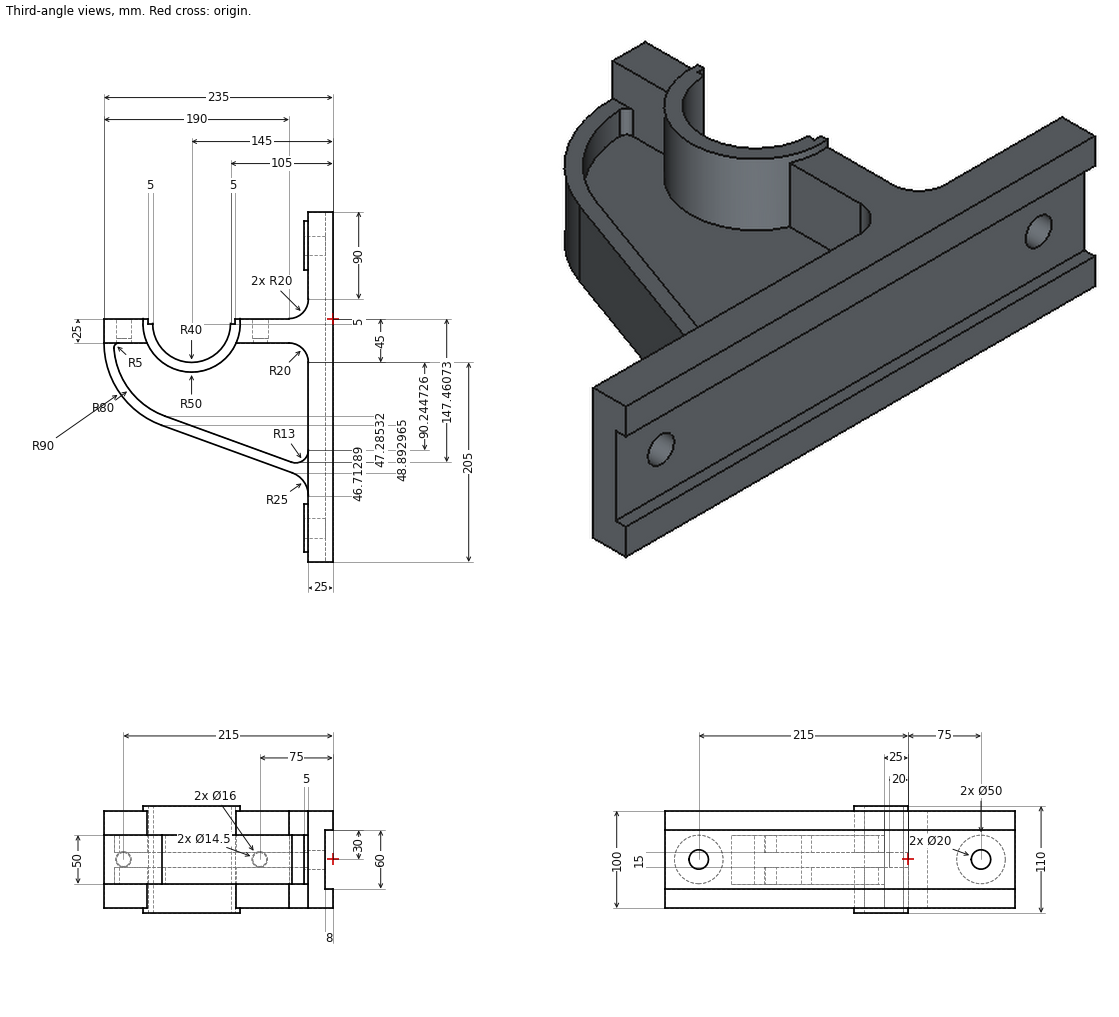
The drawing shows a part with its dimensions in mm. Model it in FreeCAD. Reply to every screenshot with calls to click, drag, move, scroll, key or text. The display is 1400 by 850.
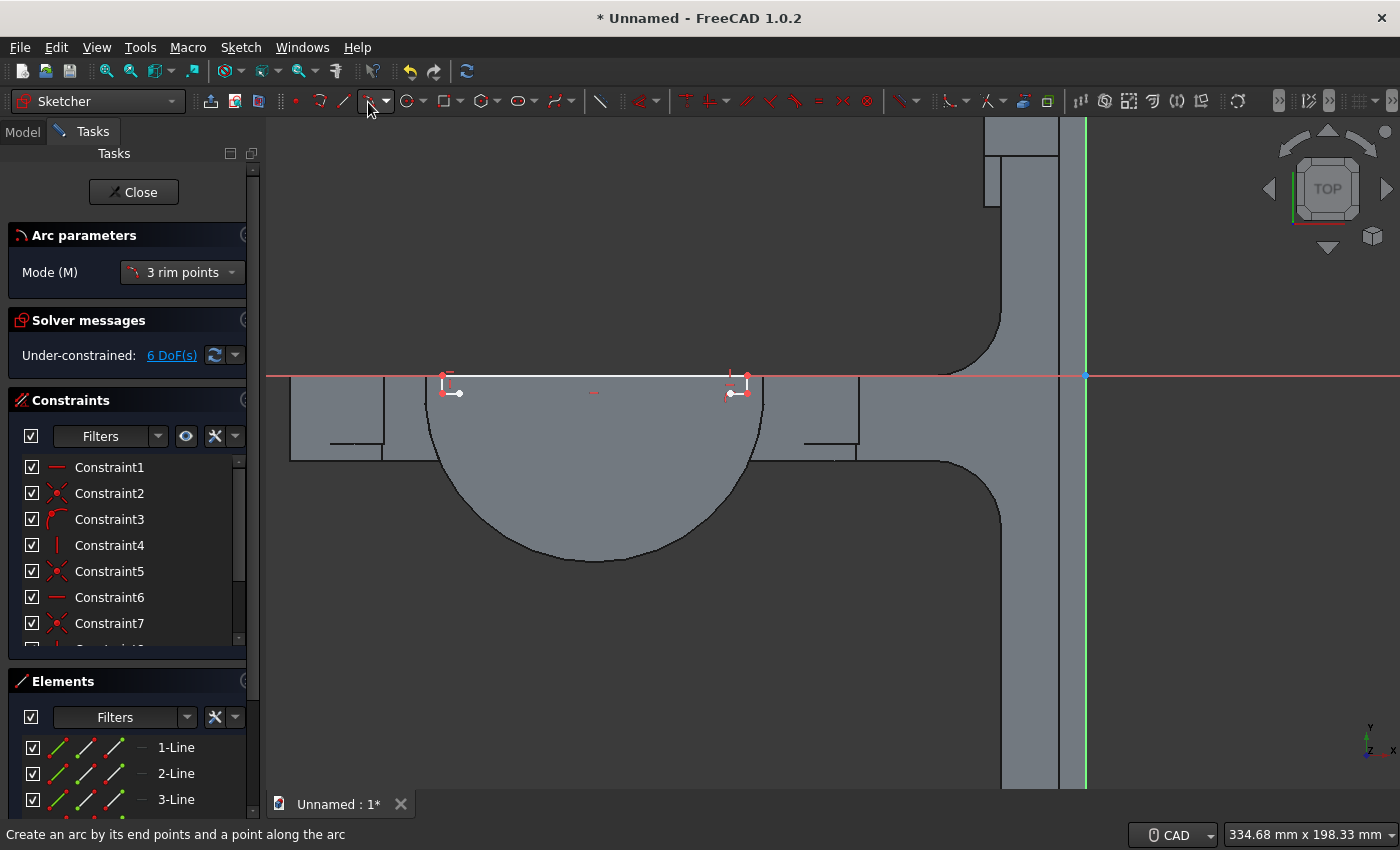
scroll(459, 393, up, 4)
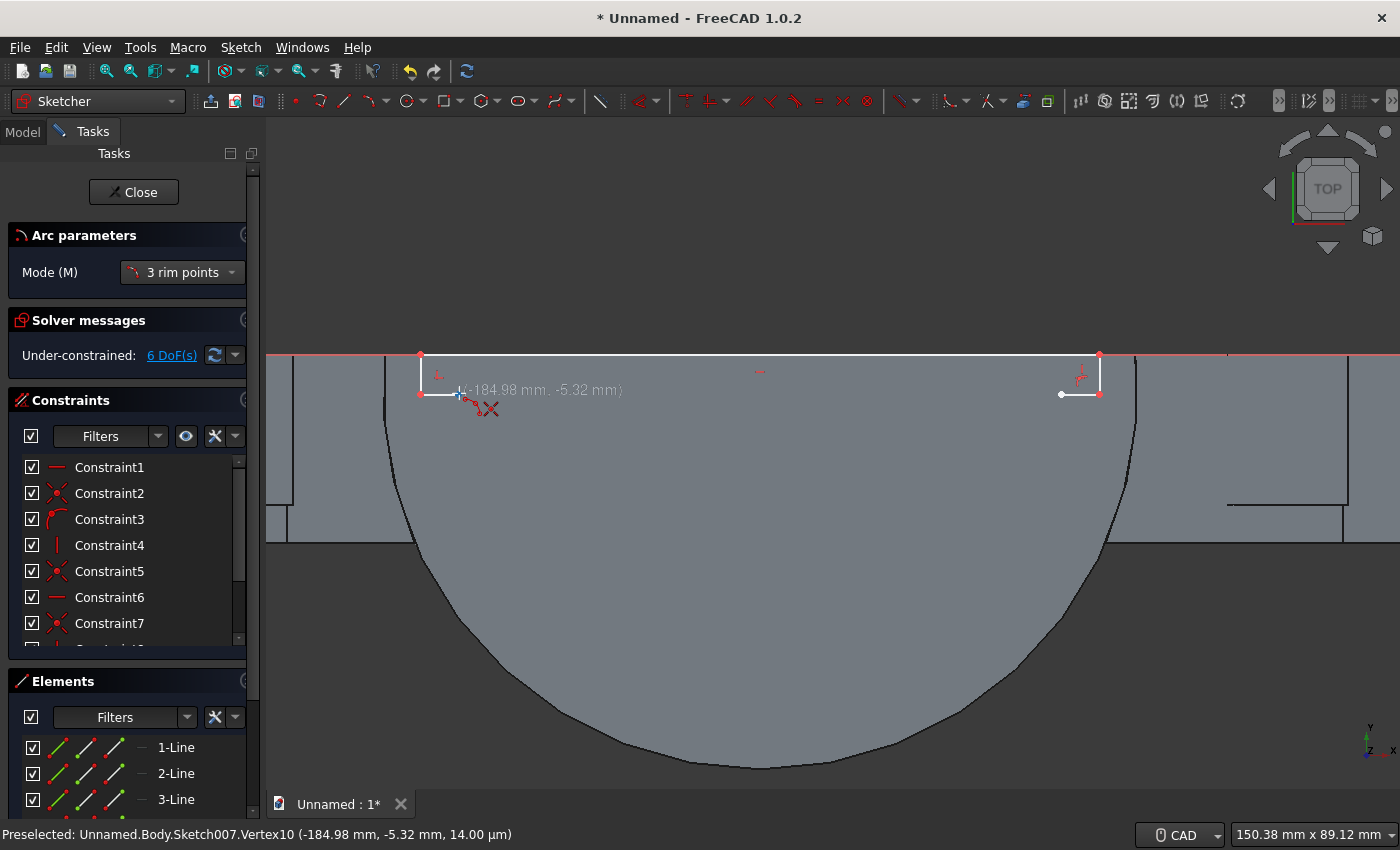
click(459, 395)
click(1062, 395)
click(760, 694)
key(Escape)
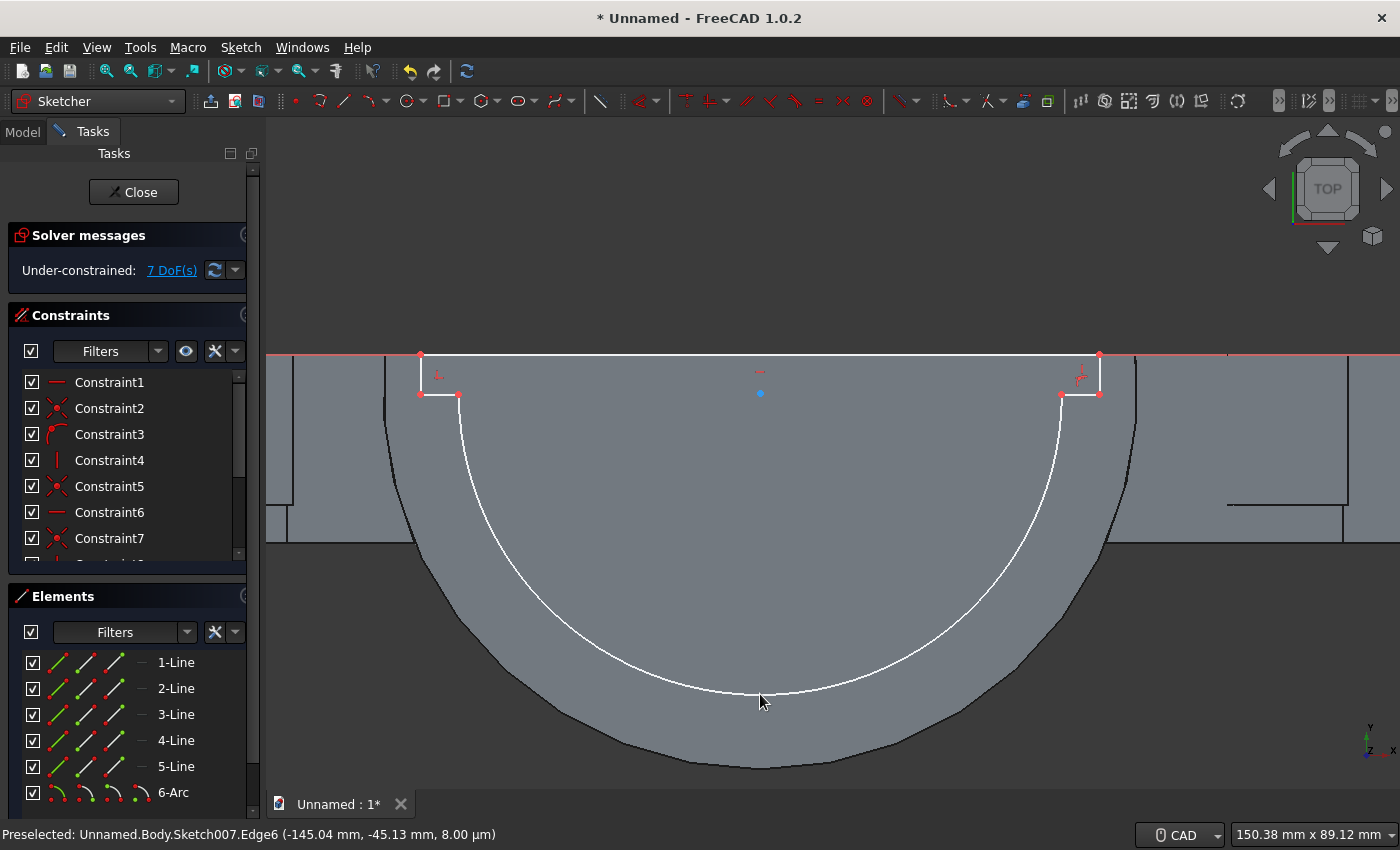
click(640, 102)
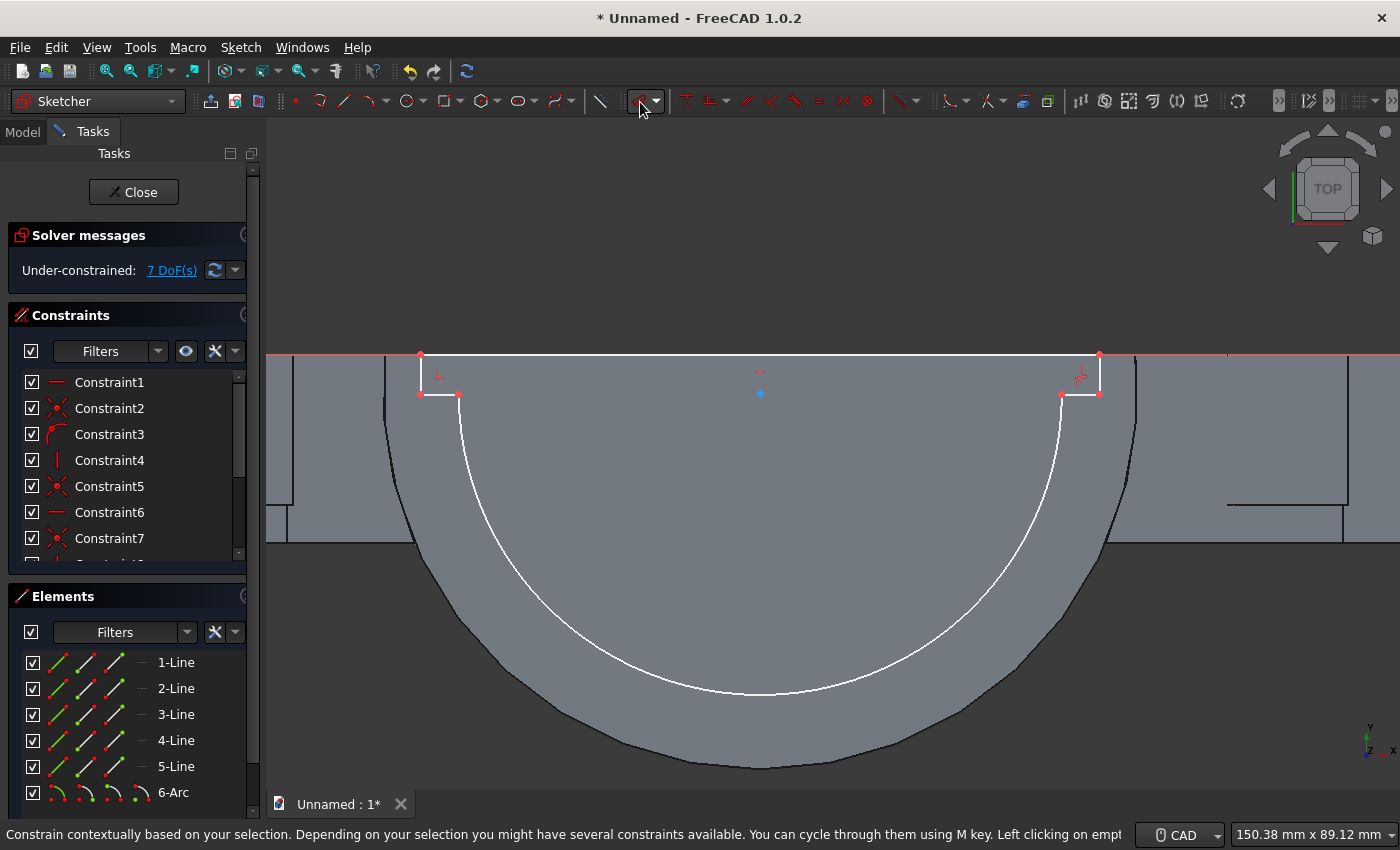
click(584, 638)
click(565, 664)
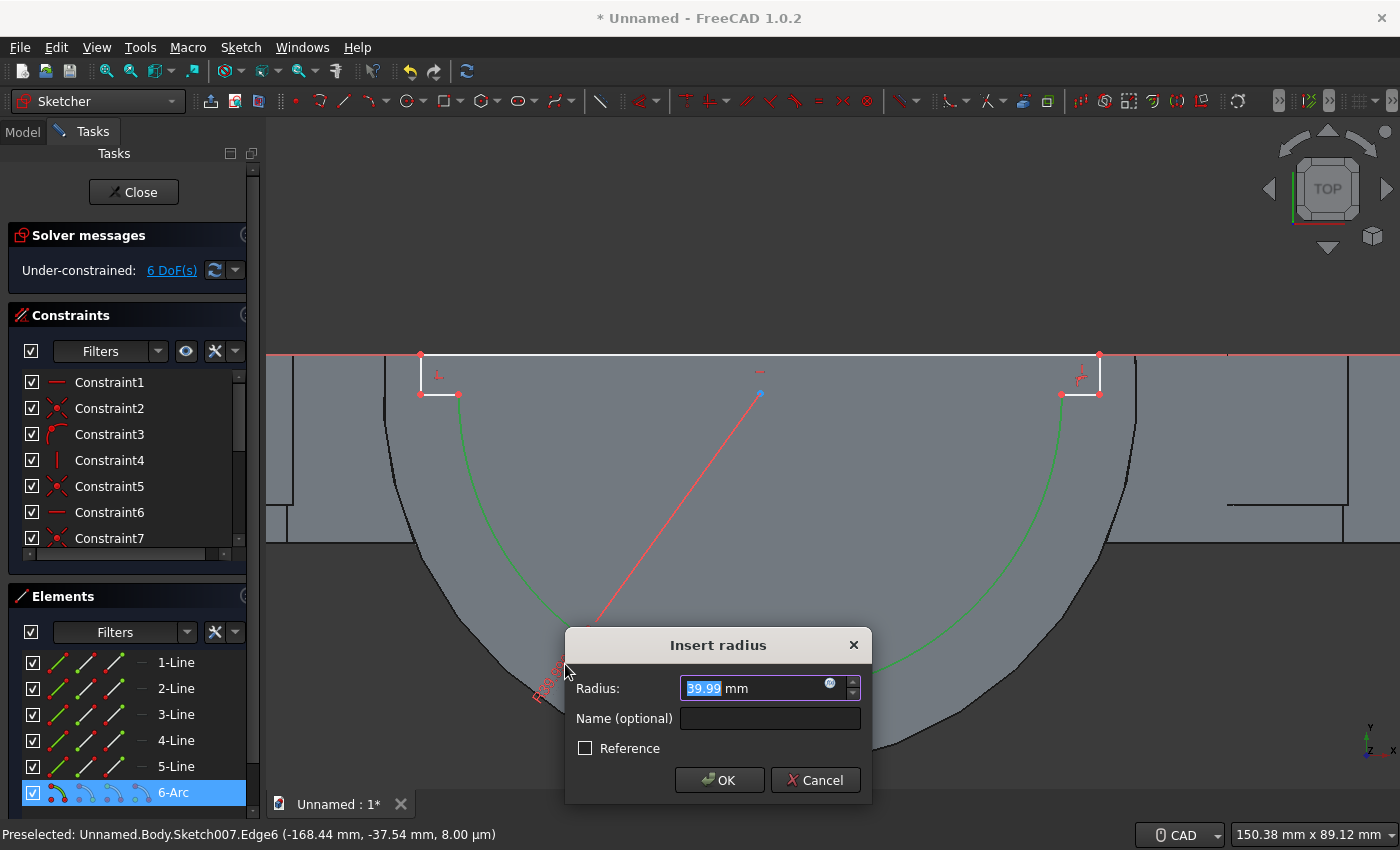
text(40)
key(Return)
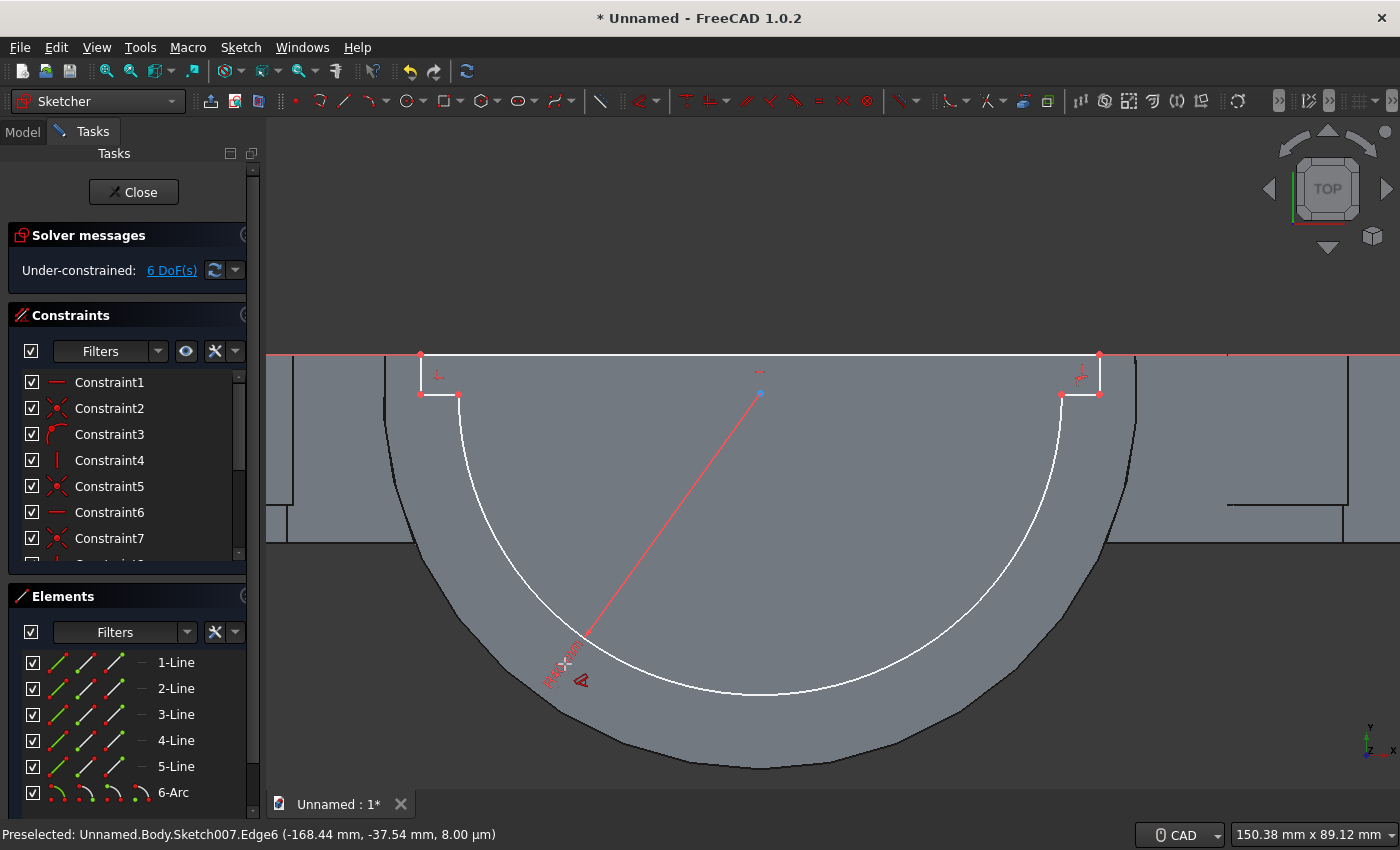
click(1073, 395)
click(1081, 429)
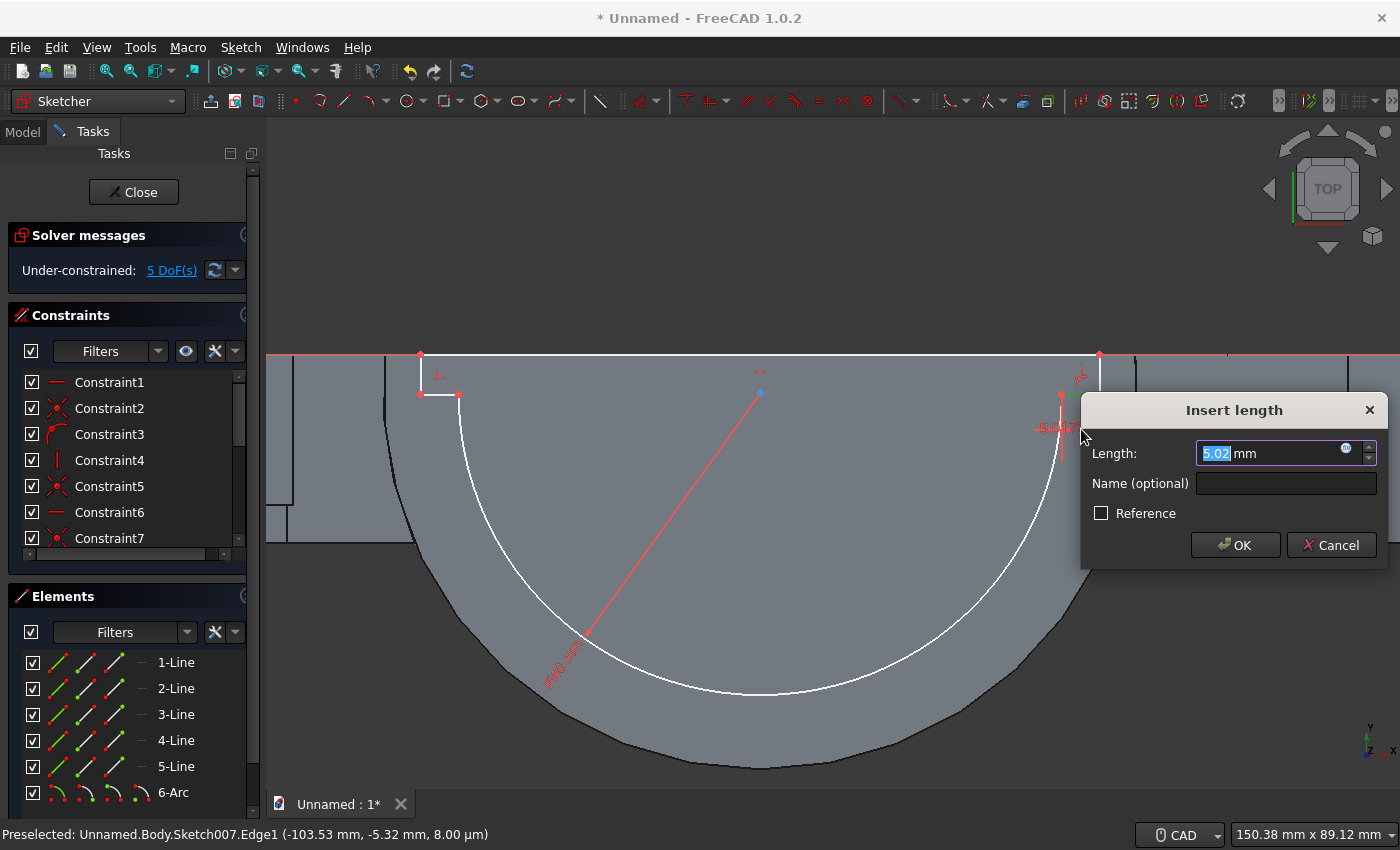
text(5)
key(Return)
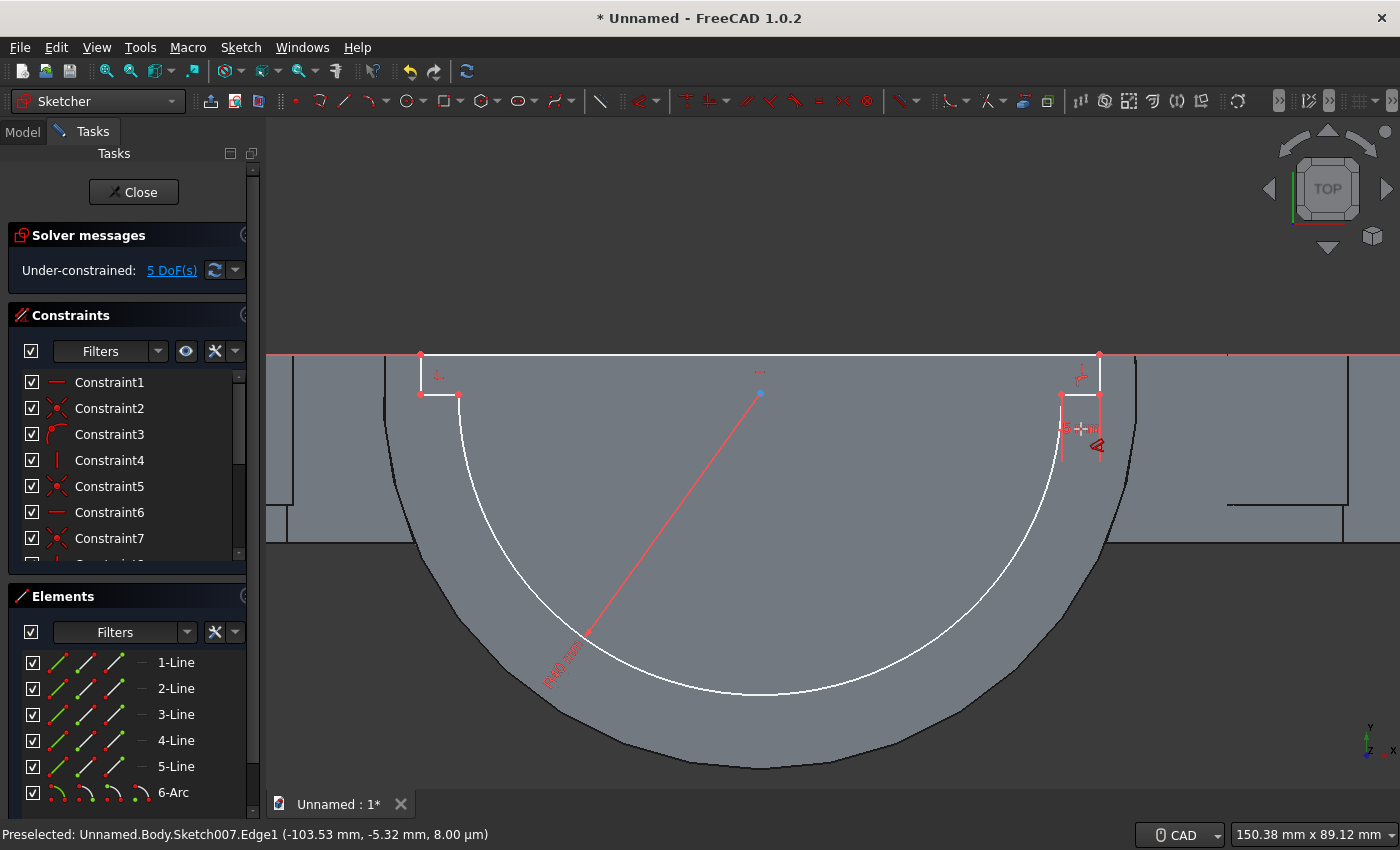
click(1100, 383)
click(1066, 375)